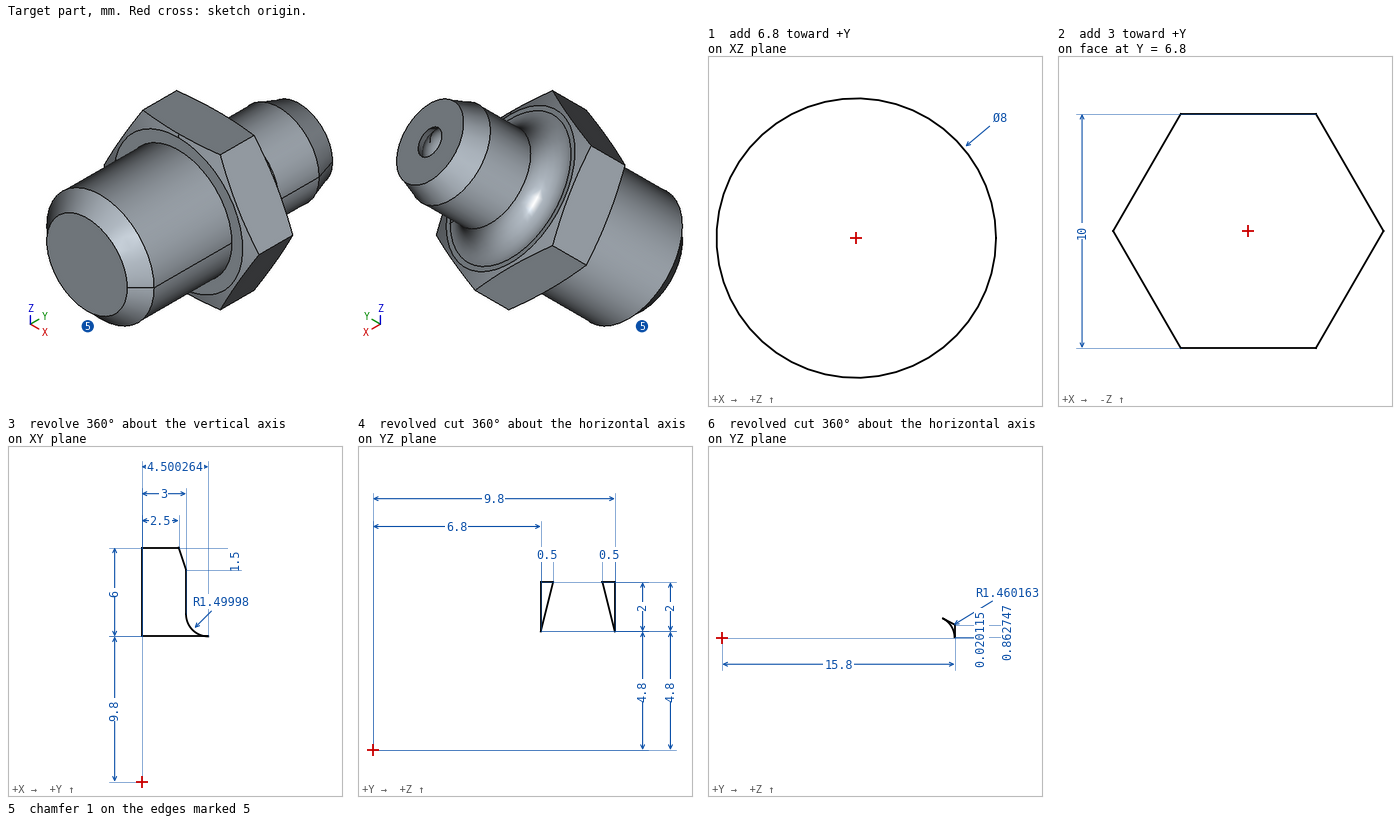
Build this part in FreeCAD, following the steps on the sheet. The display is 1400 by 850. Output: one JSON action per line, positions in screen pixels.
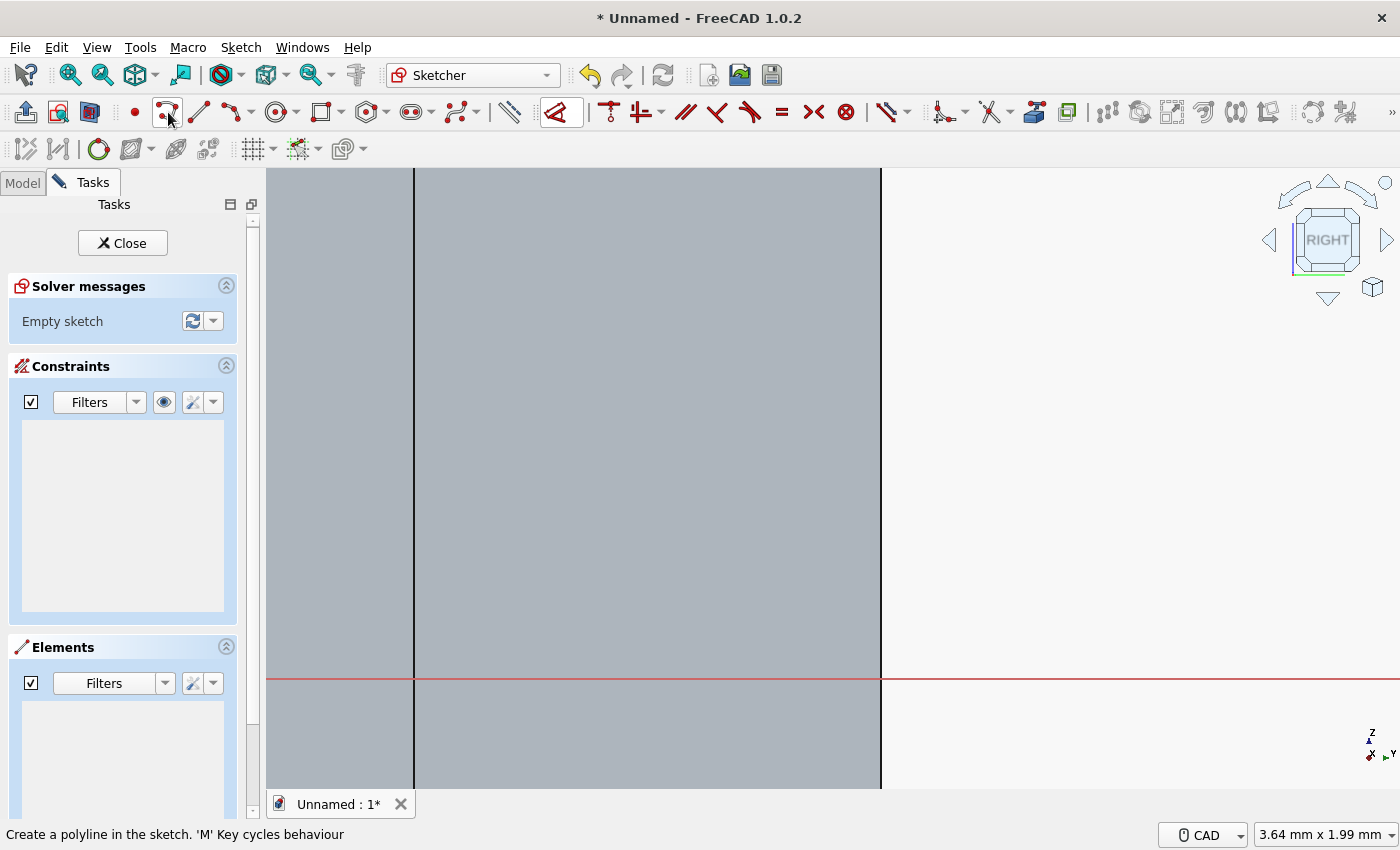
{"action": "scroll", "coordinate": [881, 673], "scroll_direction": "up", "scroll_amount": 5}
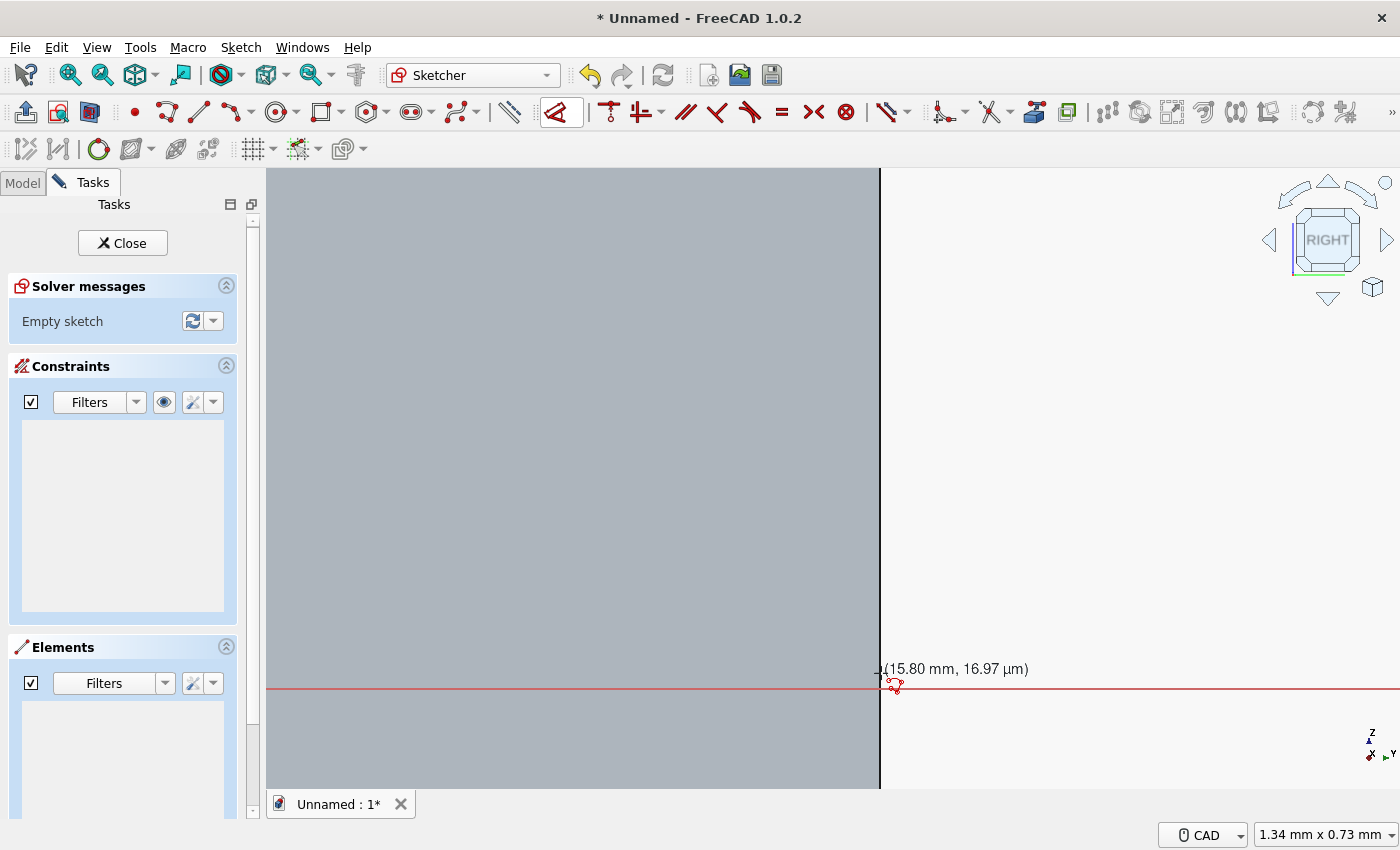
{"action": "left_click", "coordinate": [880, 672]}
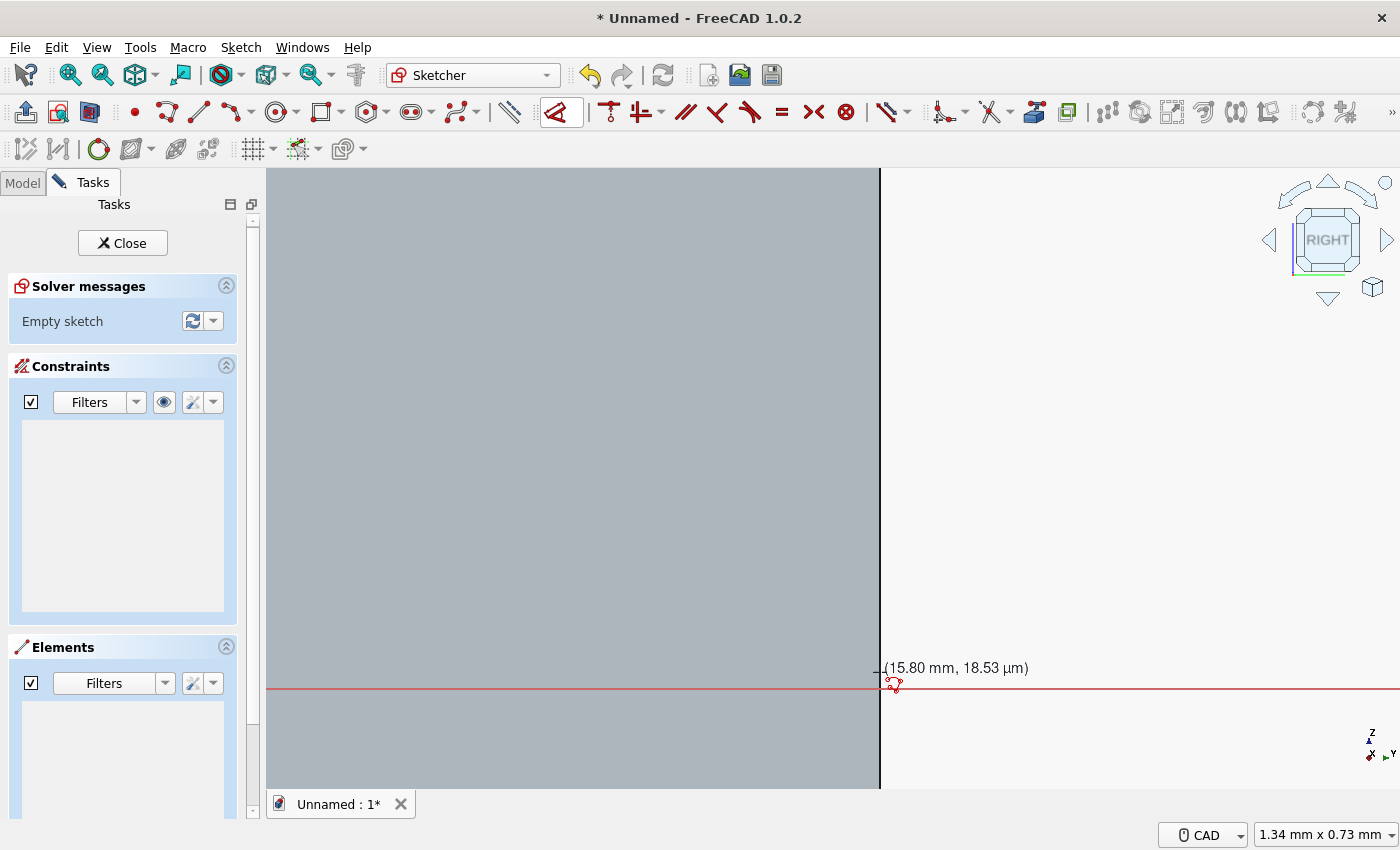
{"action": "scroll", "coordinate": [890, 680], "scroll_direction": "down", "scroll_amount": 5}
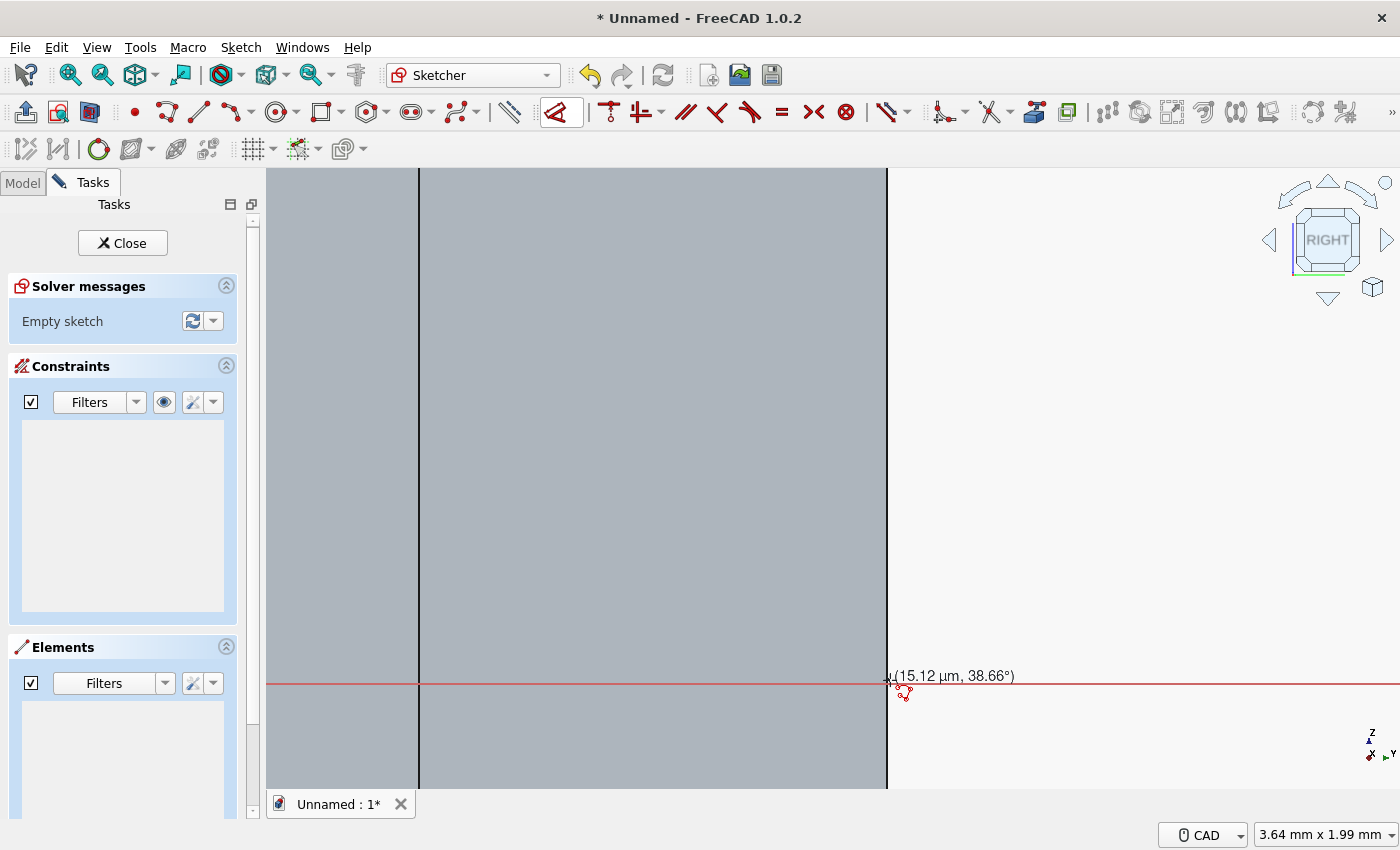
{"action": "left_click", "coordinate": [887, 409]}
{"action": "left_click", "coordinate": [643, 281]}
{"action": "right_click", "coordinate": [643, 281]}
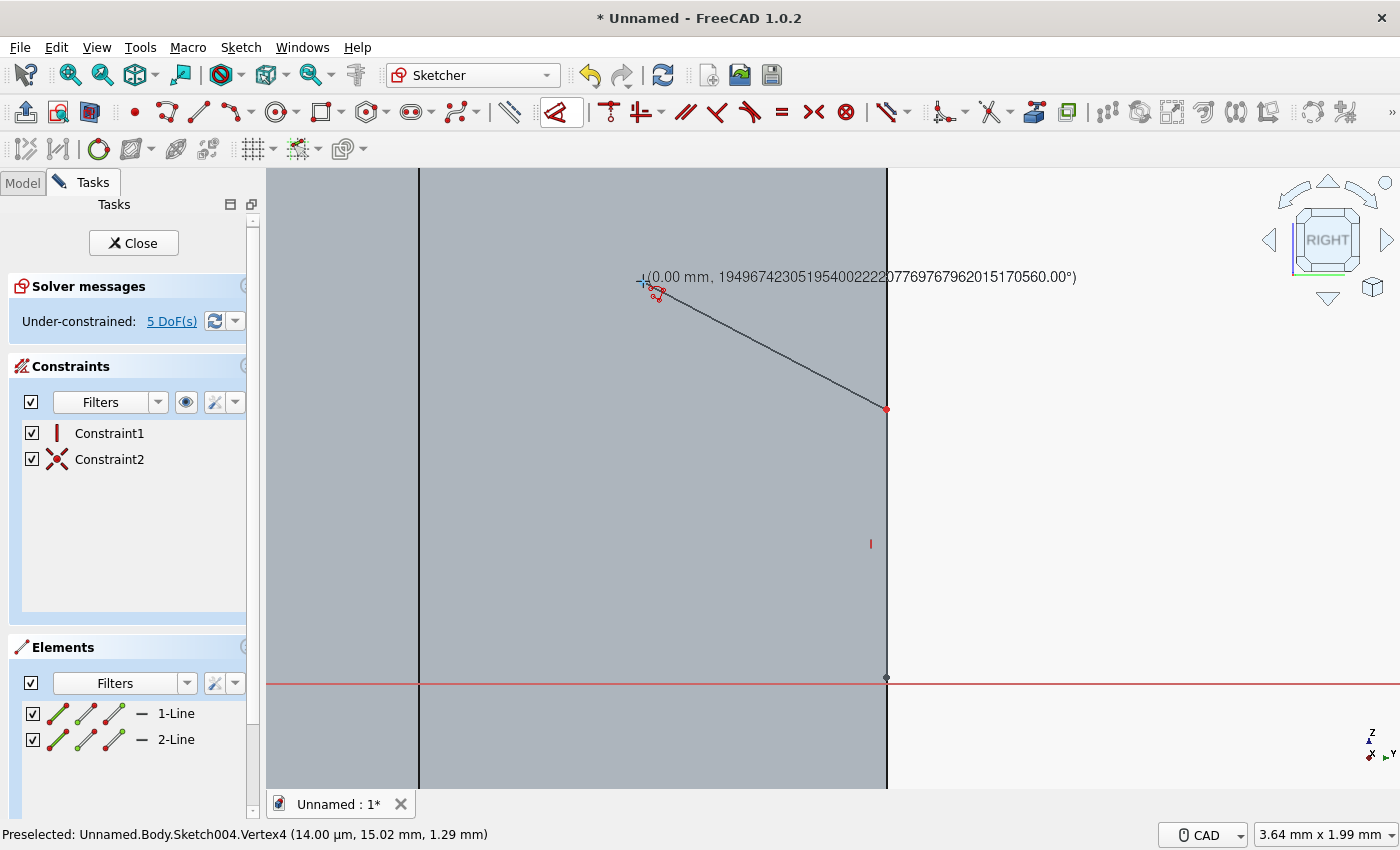
{"action": "left_click", "coordinate": [232, 112]}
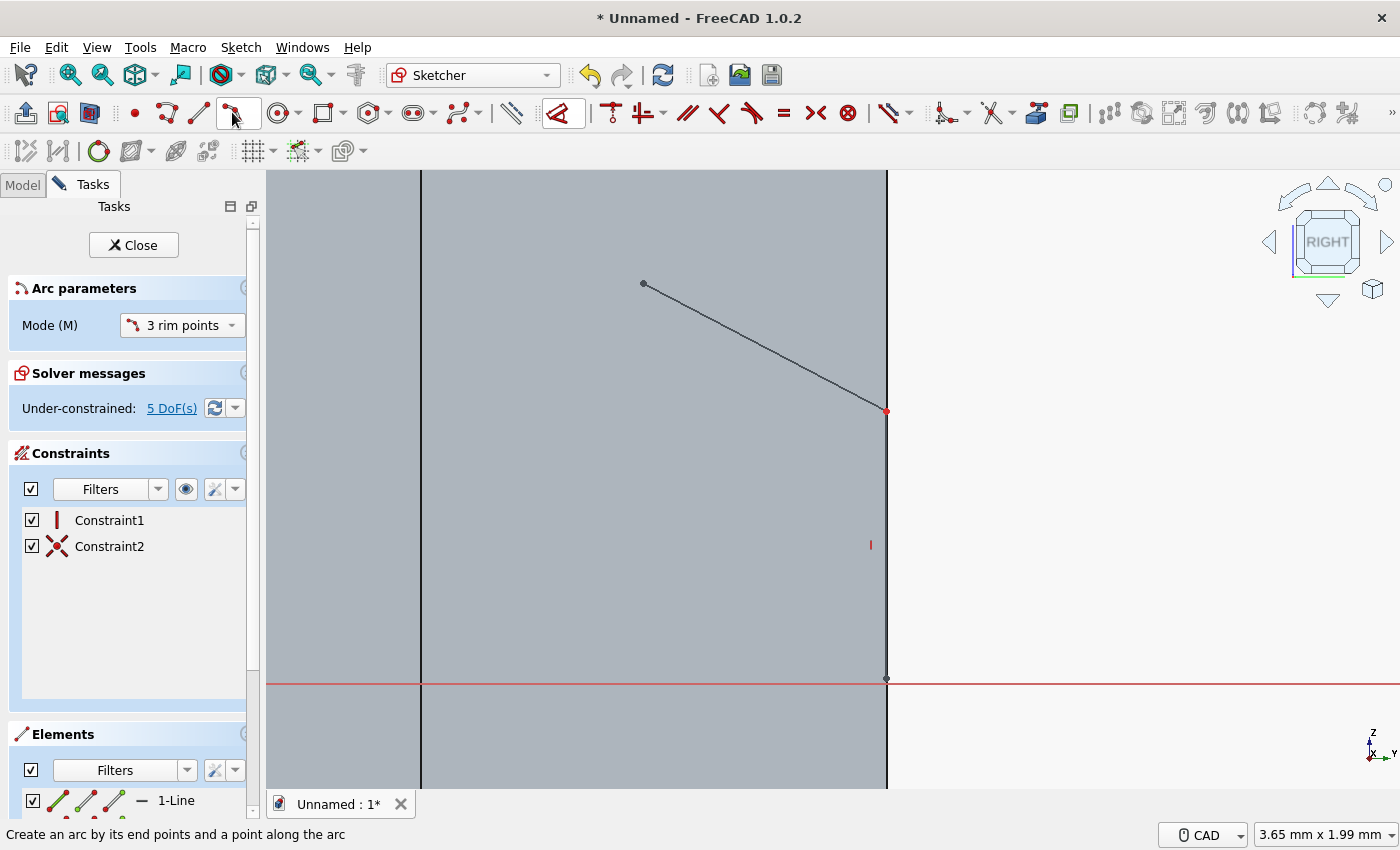
{"action": "left_click", "coordinate": [644, 284]}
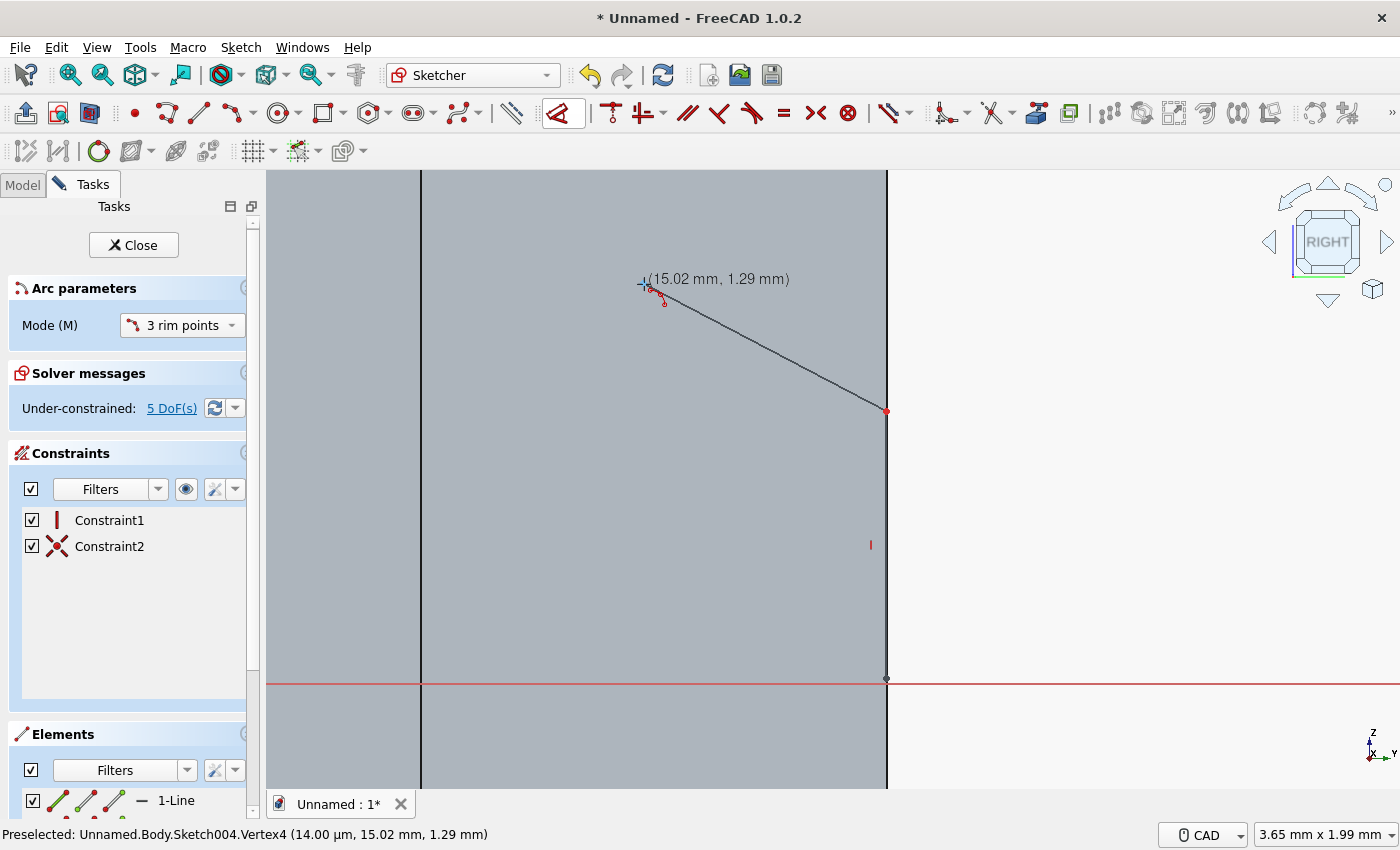
{"action": "scroll", "coordinate": [887, 678], "scroll_direction": "up", "scroll_amount": 5}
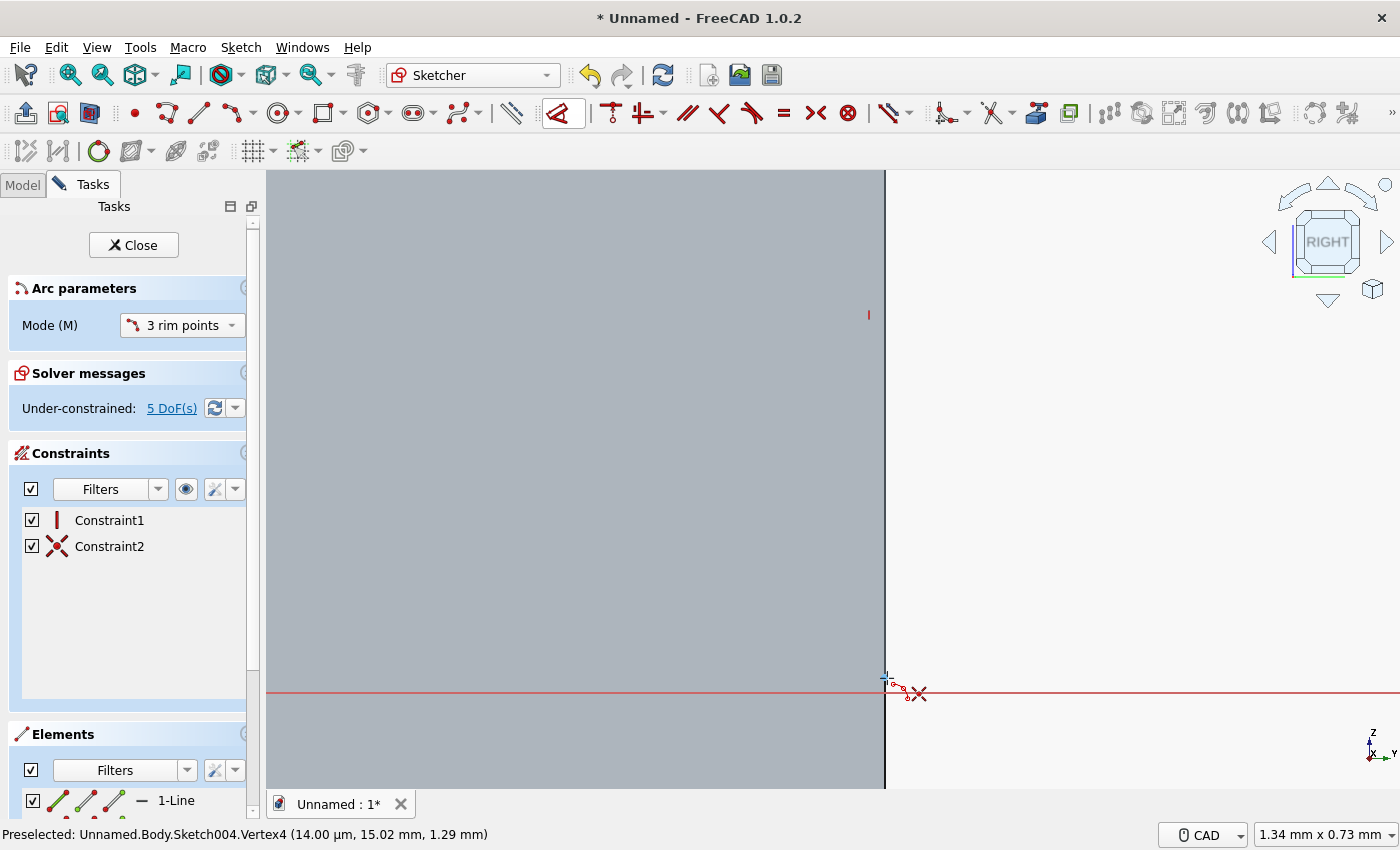
{"action": "left_click", "coordinate": [885, 677]}